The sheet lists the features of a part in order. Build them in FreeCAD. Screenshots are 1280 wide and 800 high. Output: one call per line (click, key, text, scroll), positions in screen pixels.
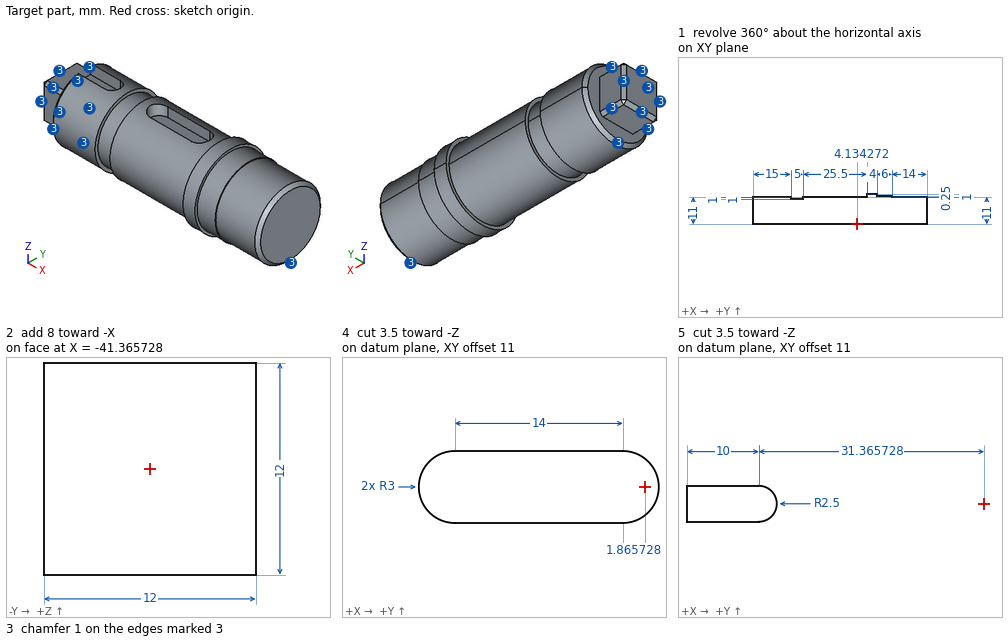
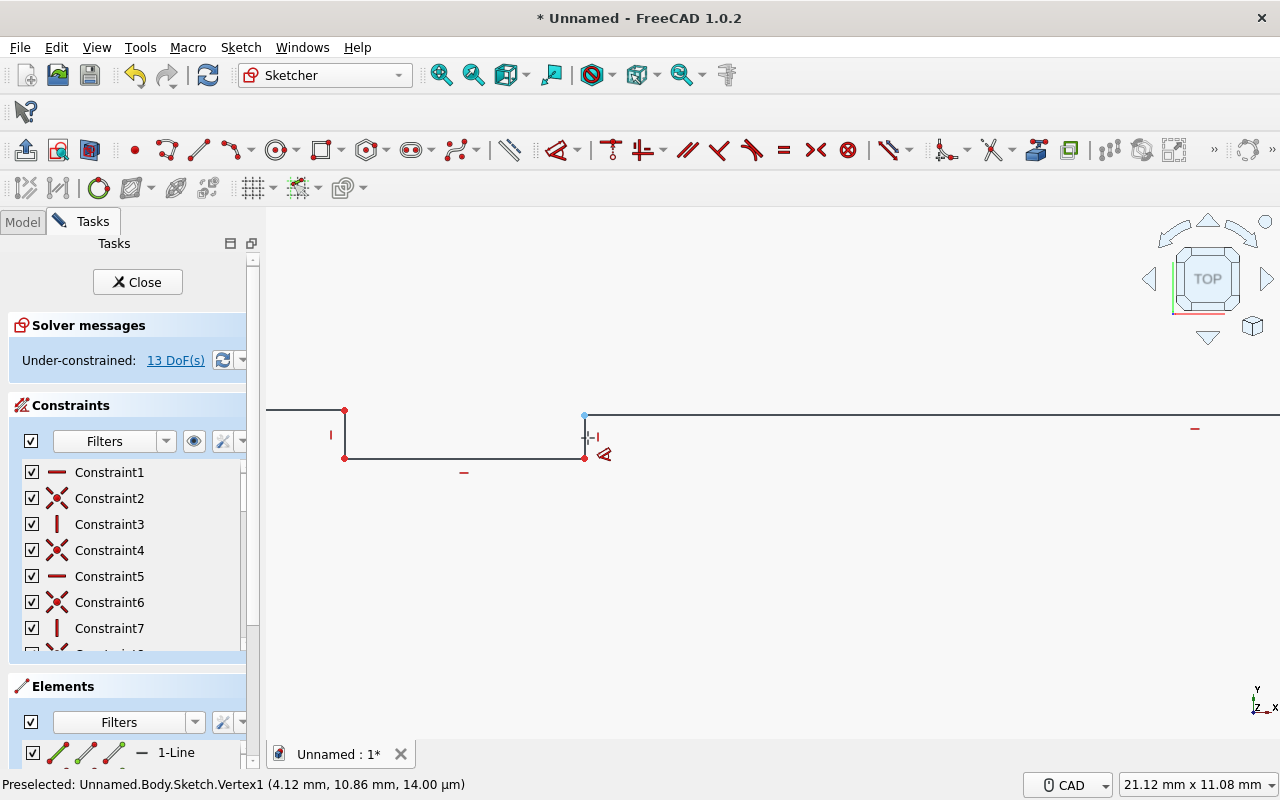
click(585, 437)
click(551, 437)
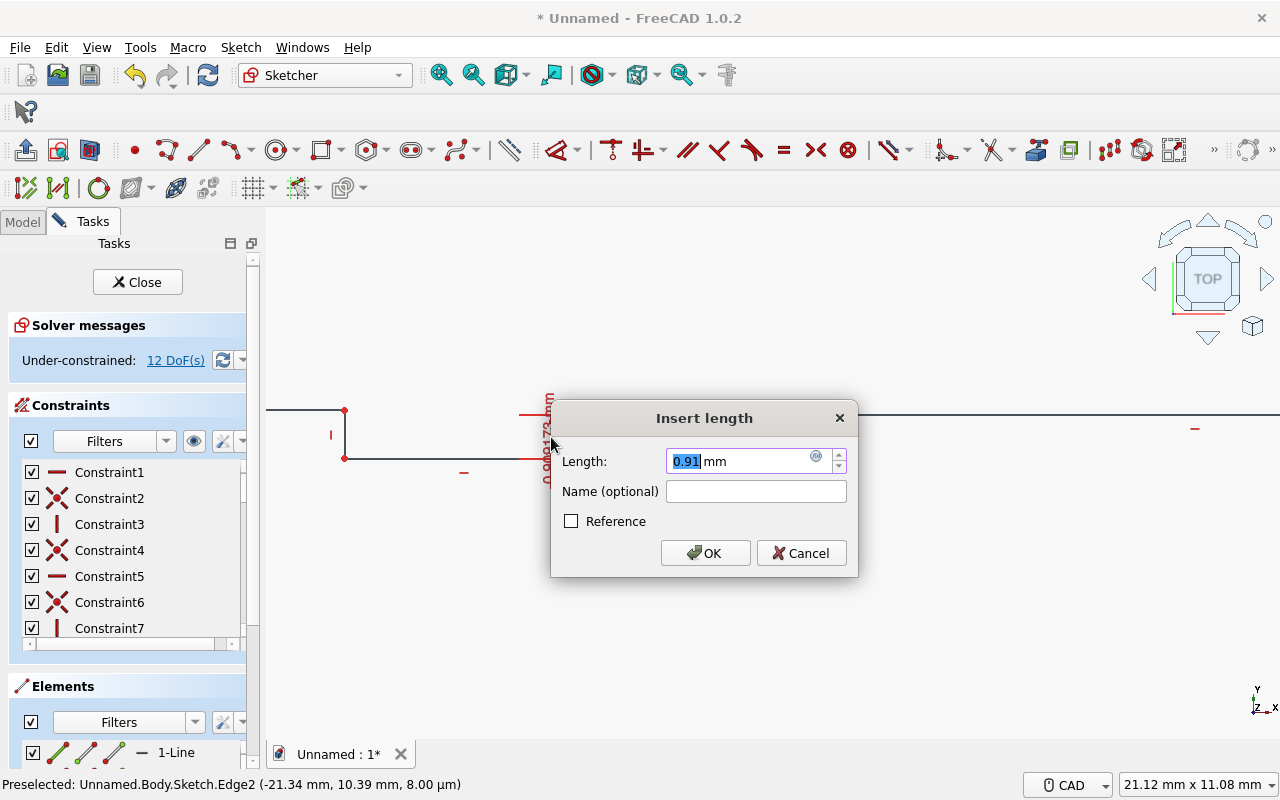
text(1)
key(Return)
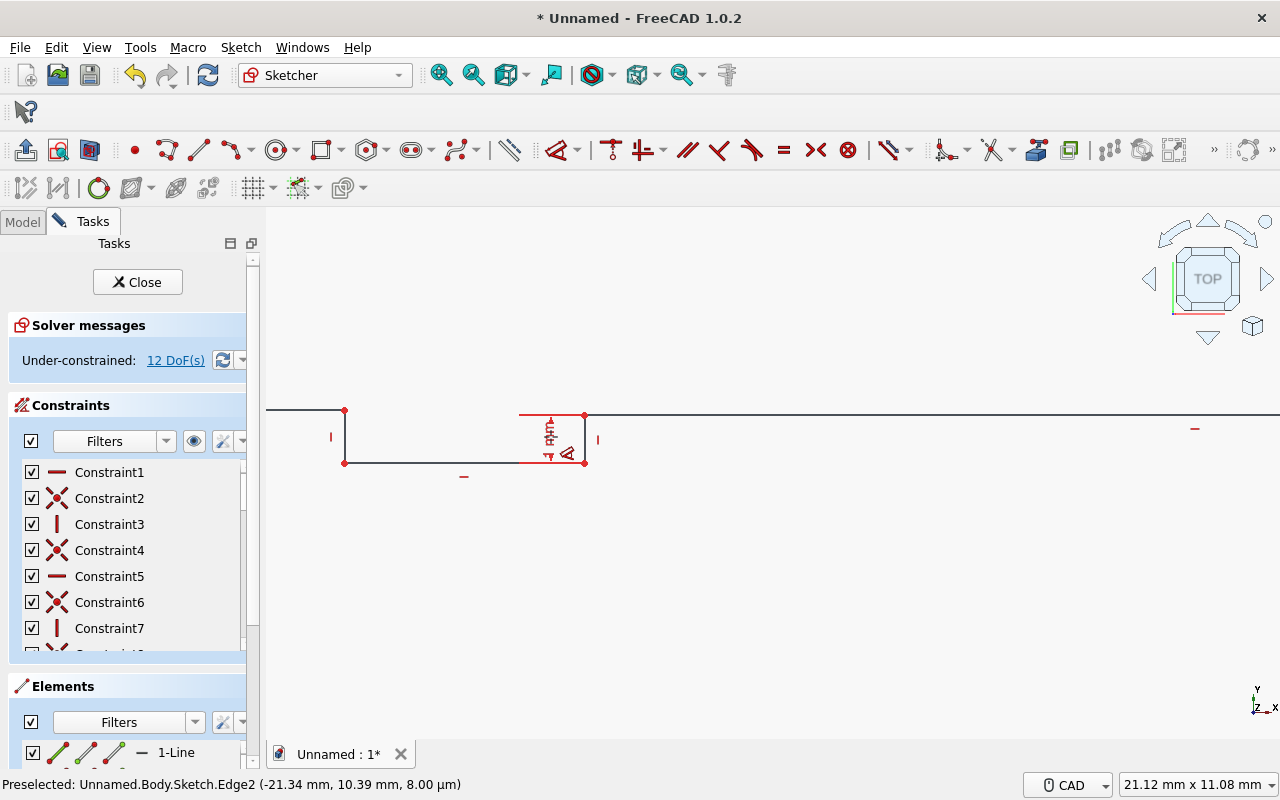
scroll(588, 438, down, 9)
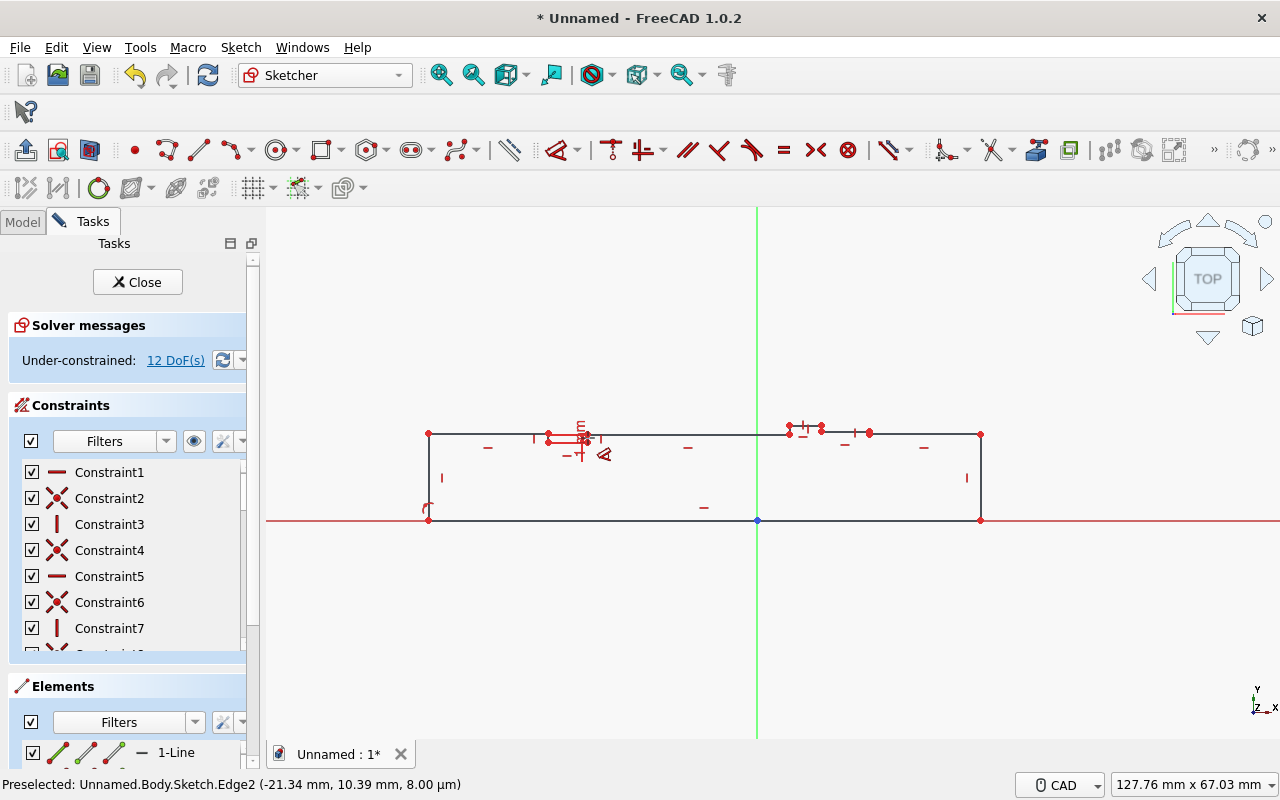
click(576, 443)
click(568, 409)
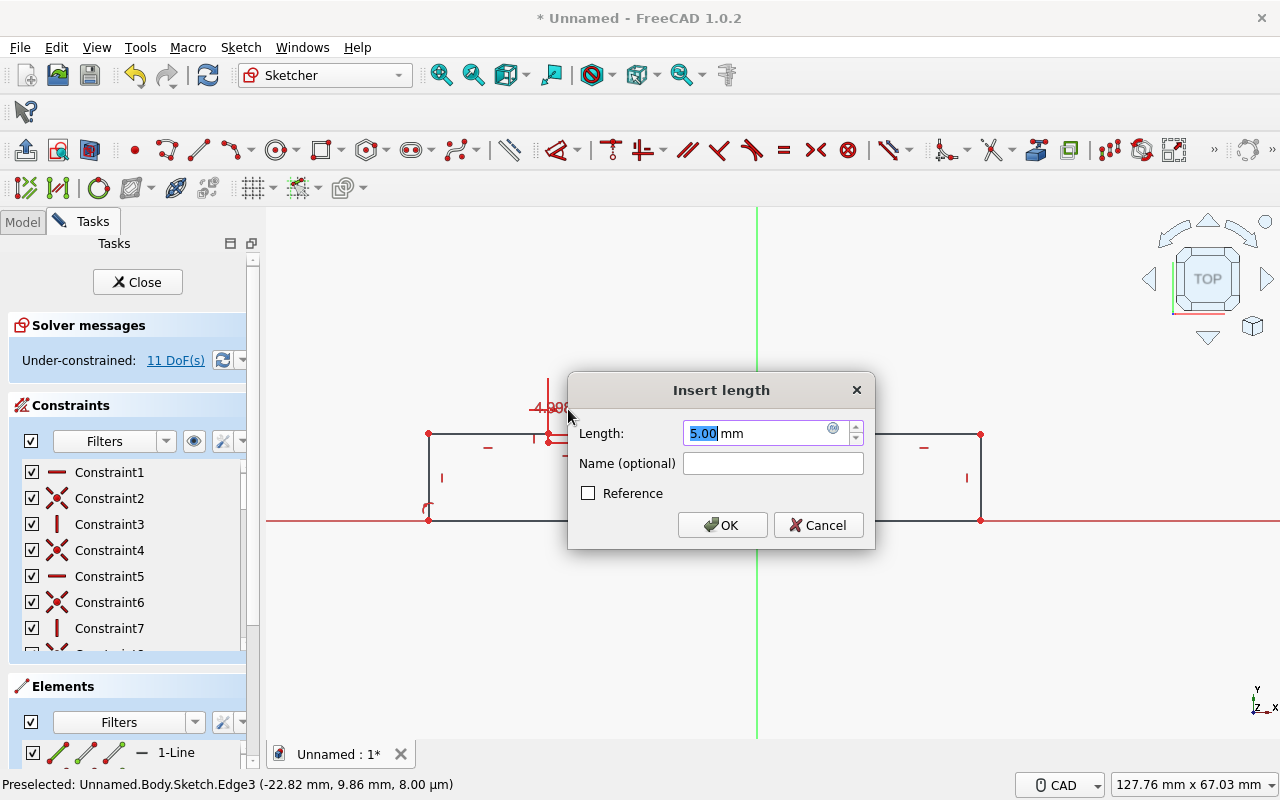
text(5)
key(Return)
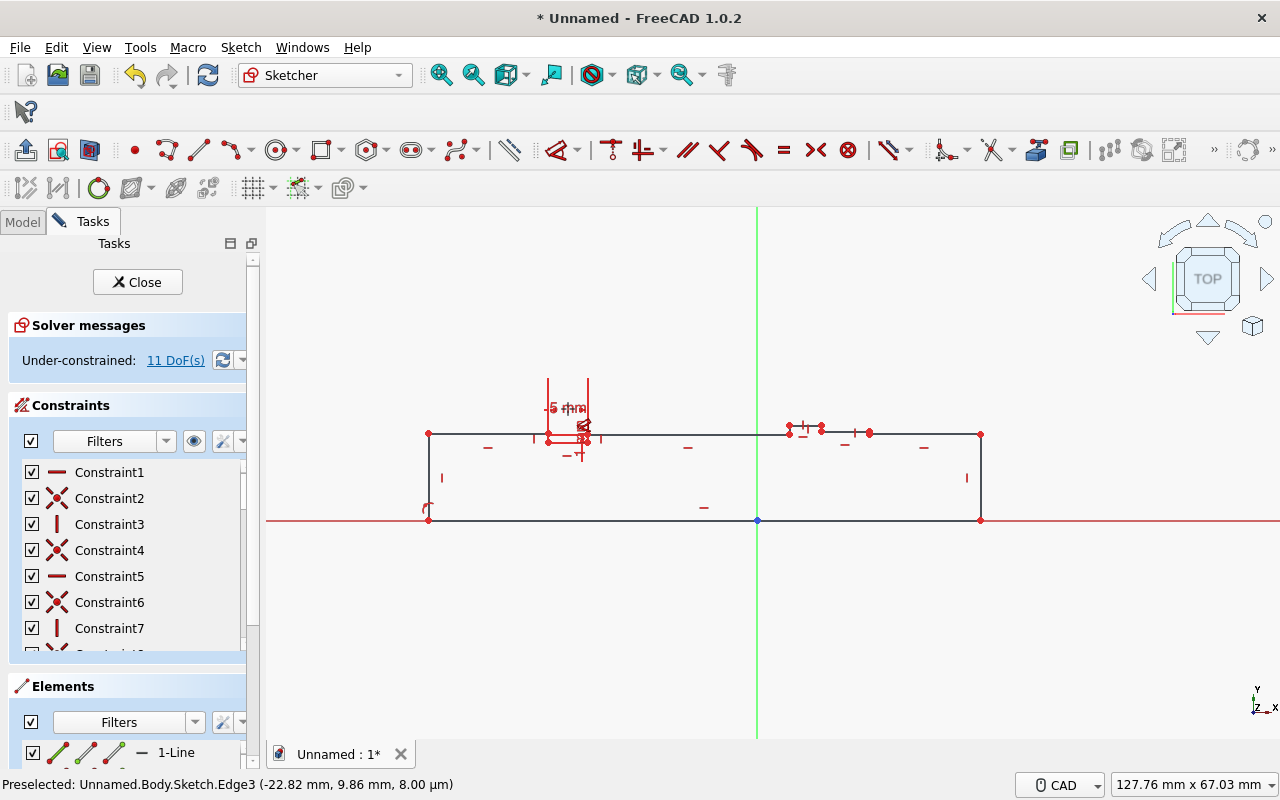
scroll(548, 438, up, 9)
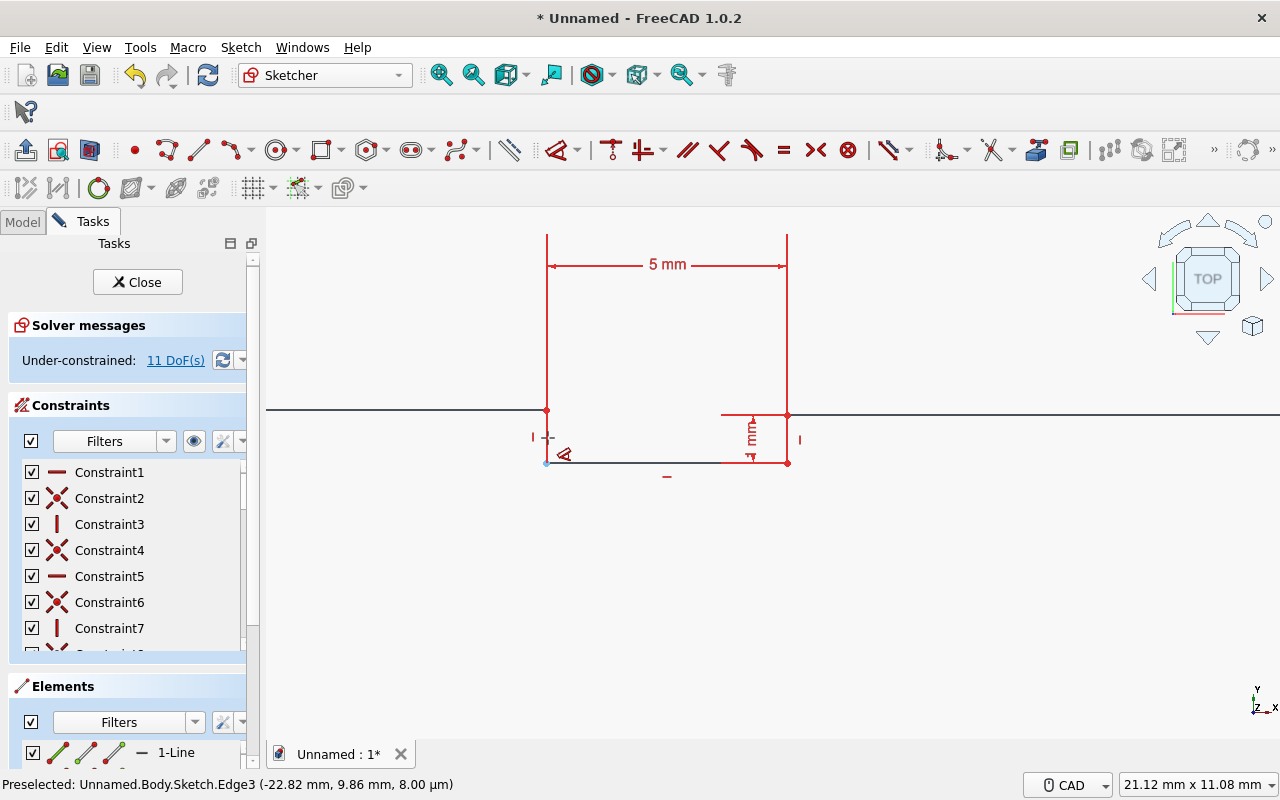
click(547, 437)
click(513, 437)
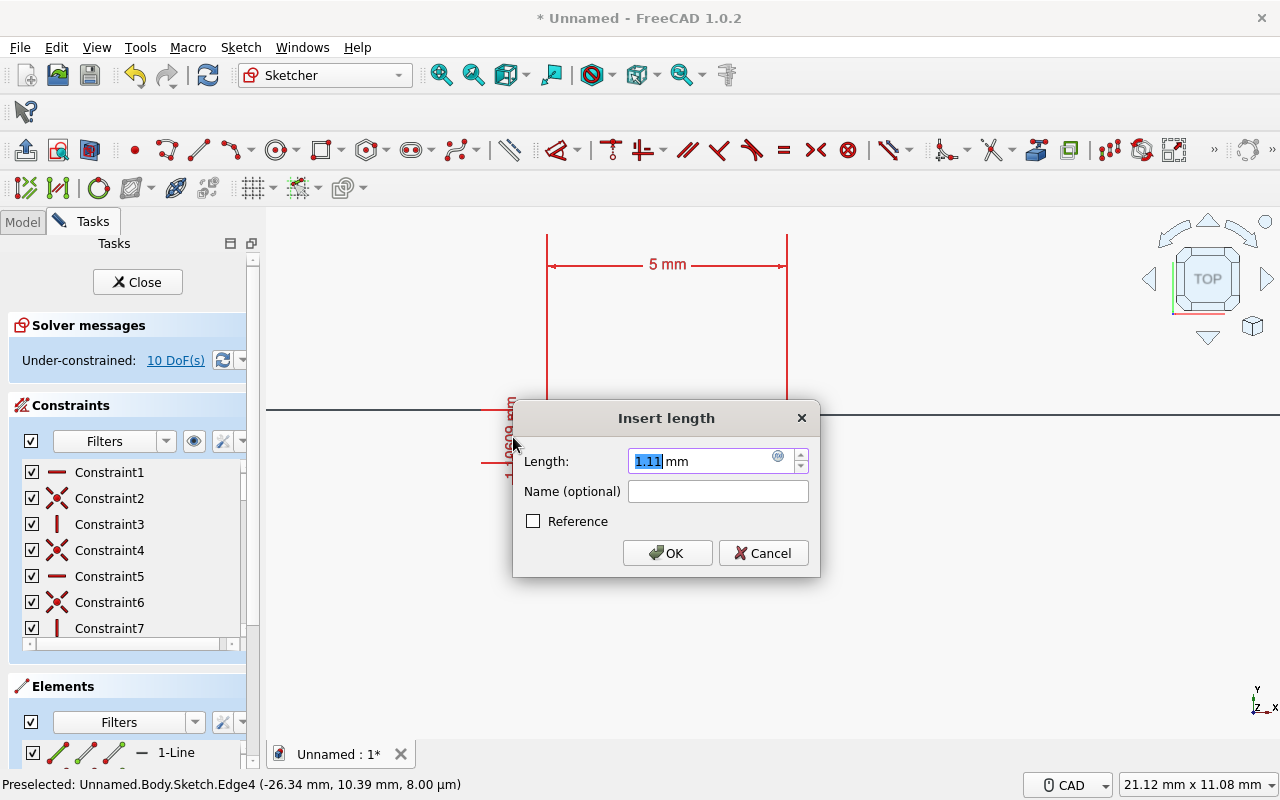
text(1)
key(Return)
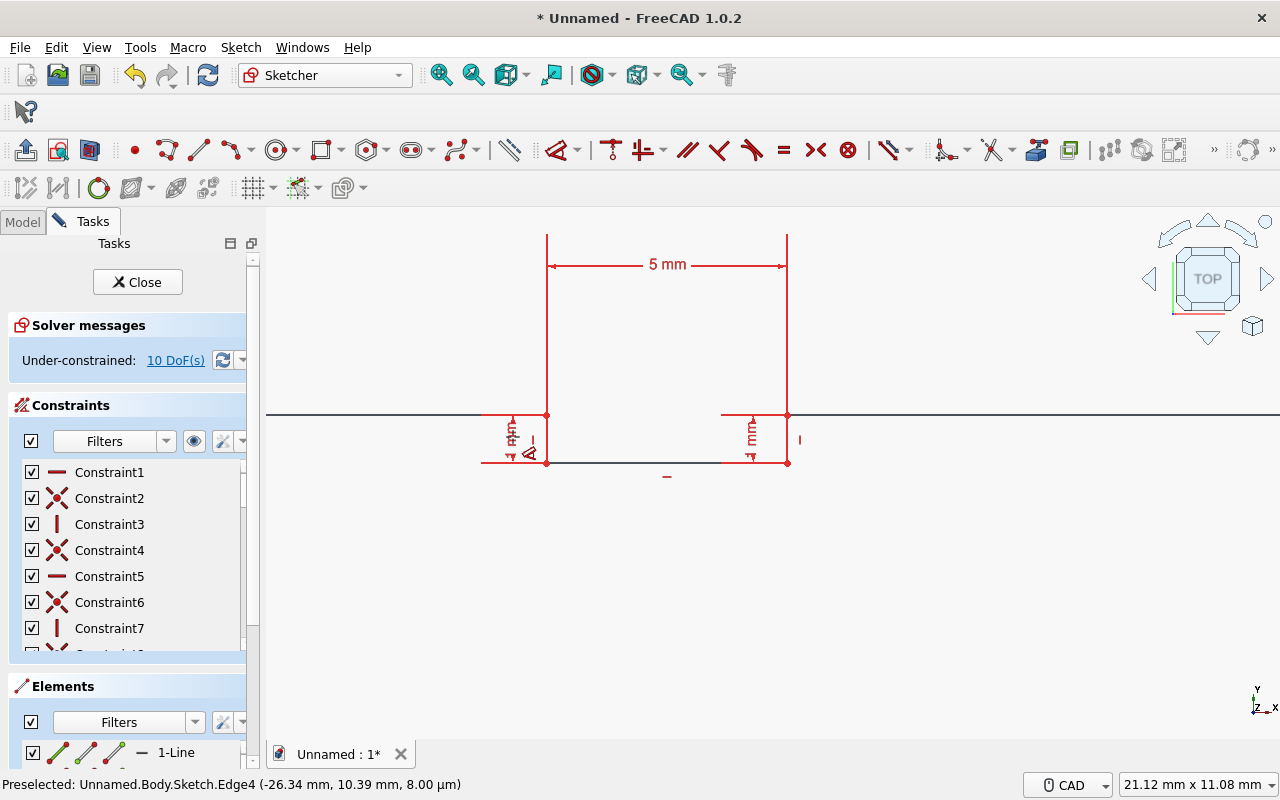
scroll(548, 438, down, 9)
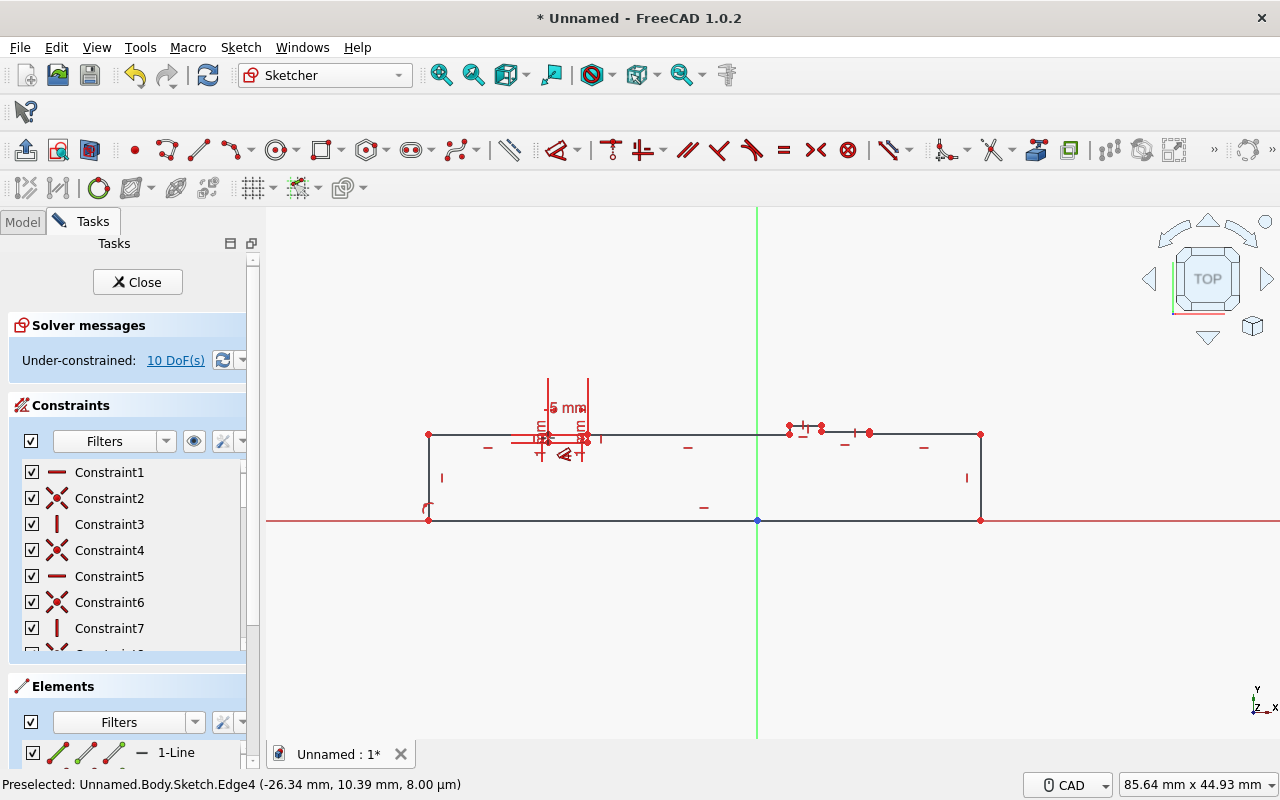
click(855, 432)
click(845, 398)